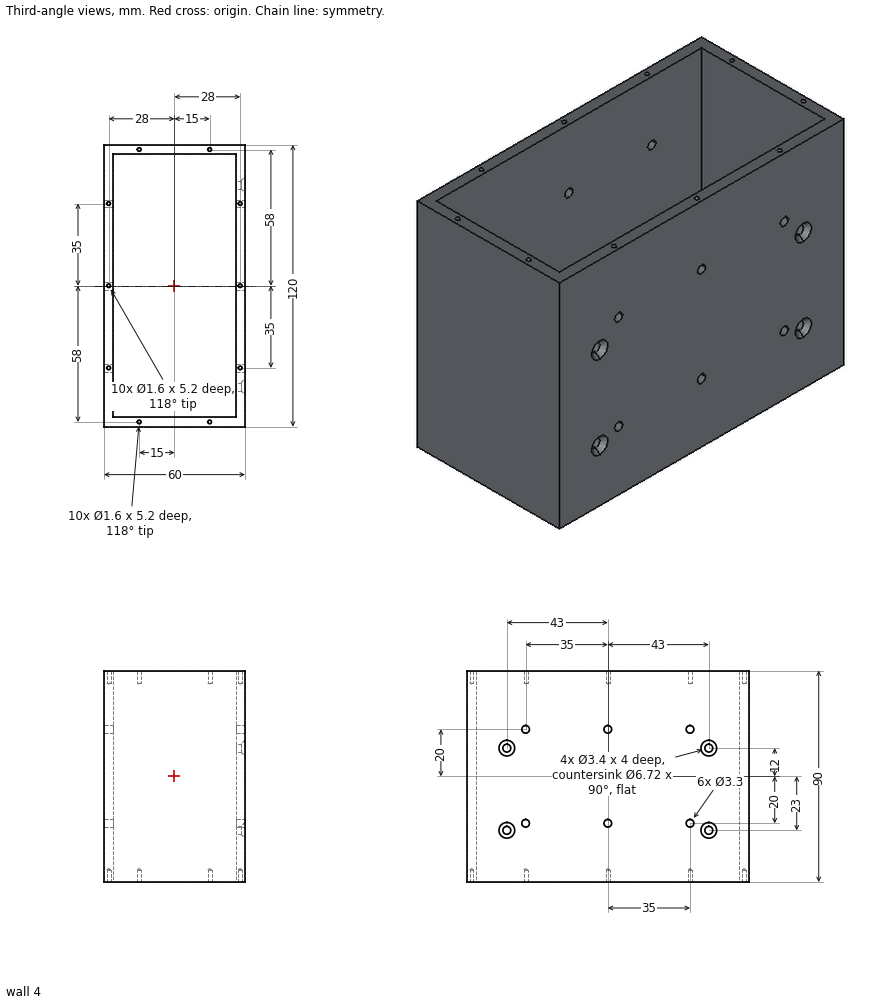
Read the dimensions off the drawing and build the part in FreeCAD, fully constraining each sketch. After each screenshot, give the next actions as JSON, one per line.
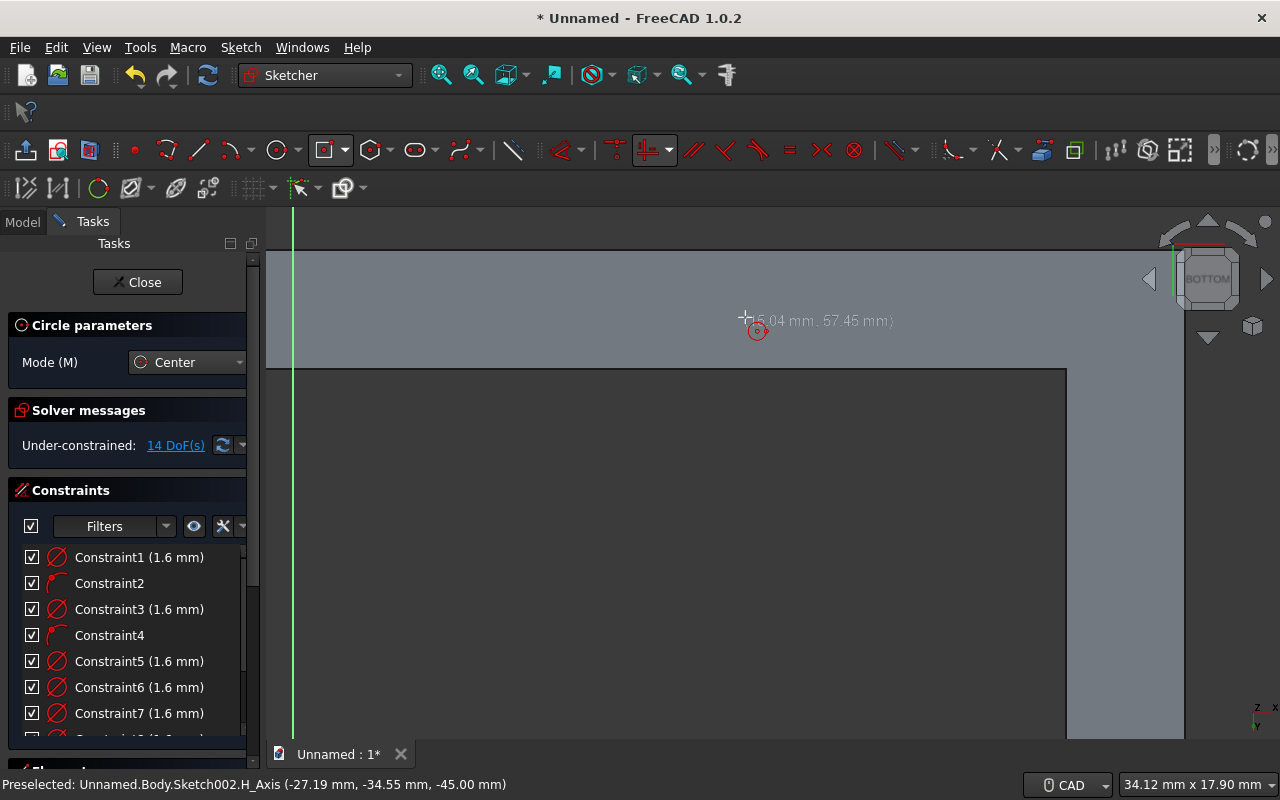
{"action": "scroll", "coordinate": [746, 317], "scroll_direction": "down", "scroll_amount": 12}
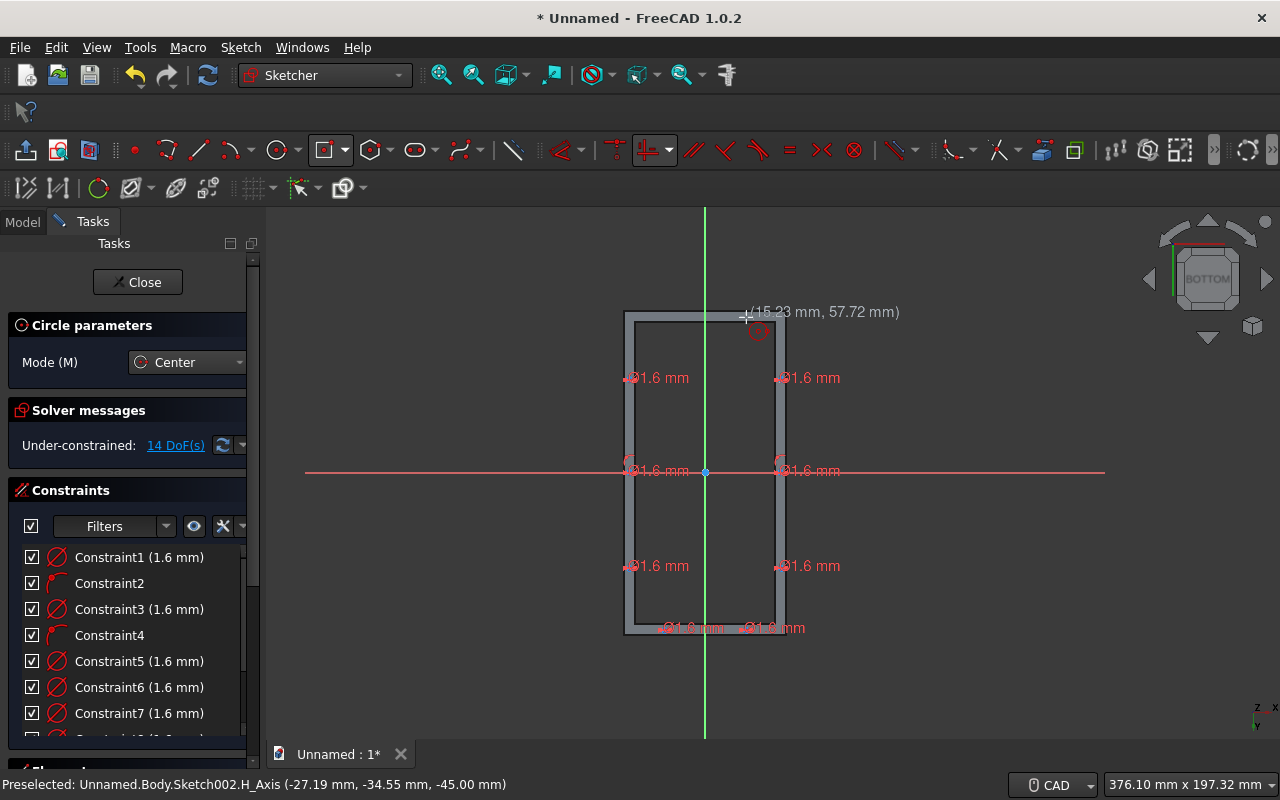
{"action": "left_click", "coordinate": [746, 317]}
{"action": "mouse_move", "coordinate": [747, 315]}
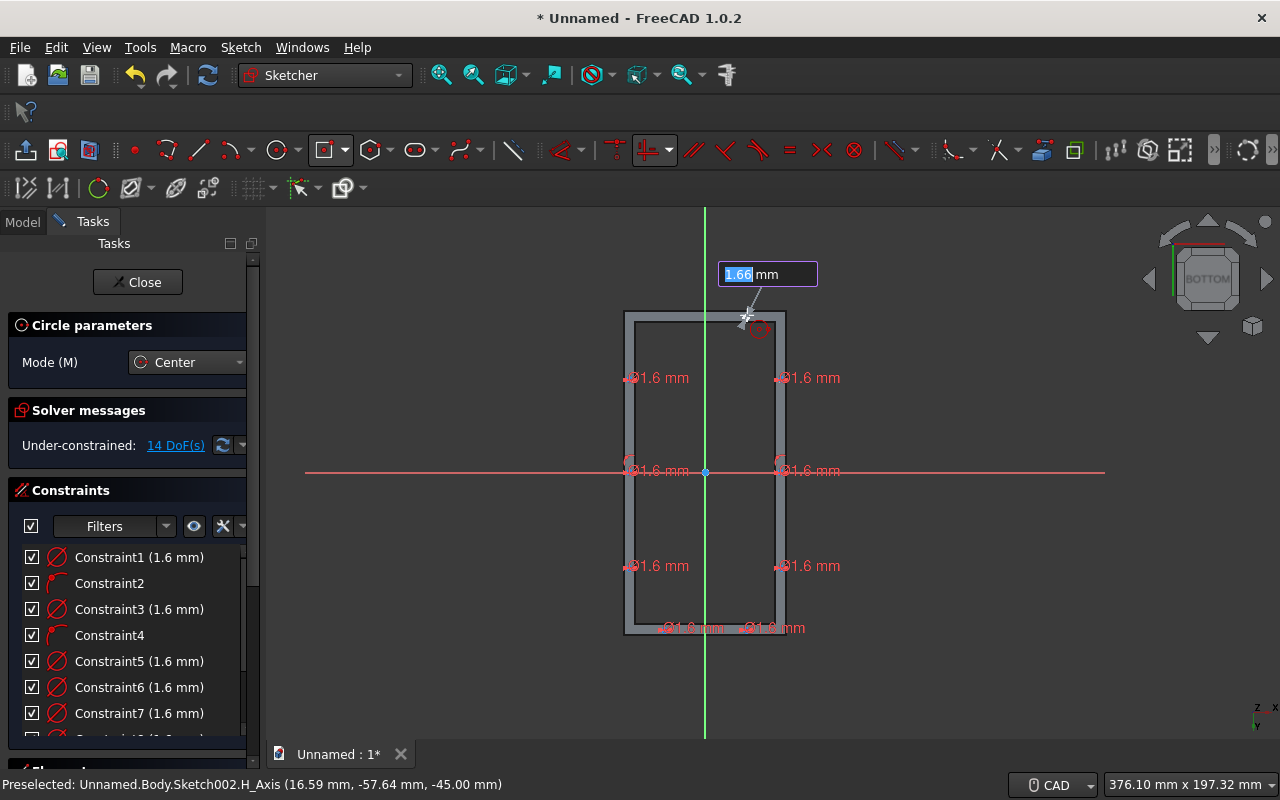
{"action": "type", "text": "1.6"}
{"action": "key", "text": "Return"}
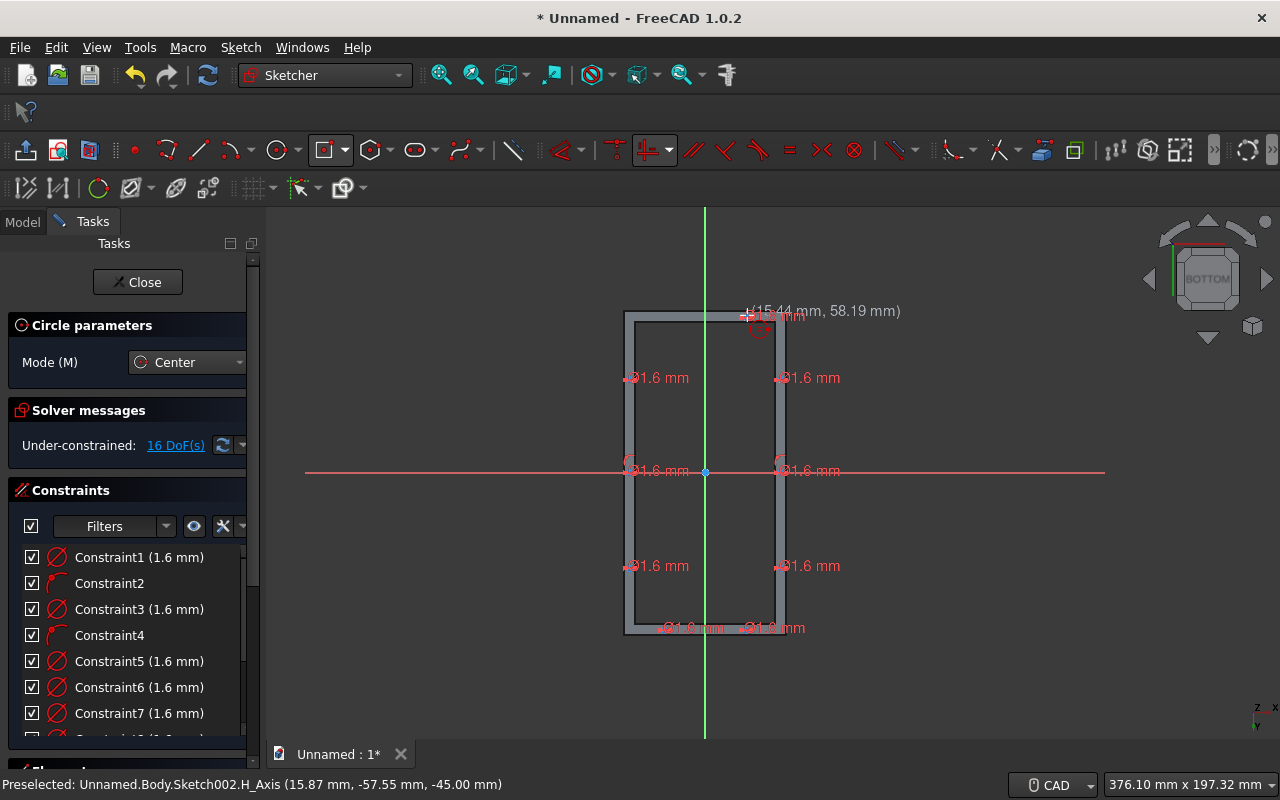
{"action": "scroll", "coordinate": [665, 317], "scroll_direction": "up", "scroll_amount": 12}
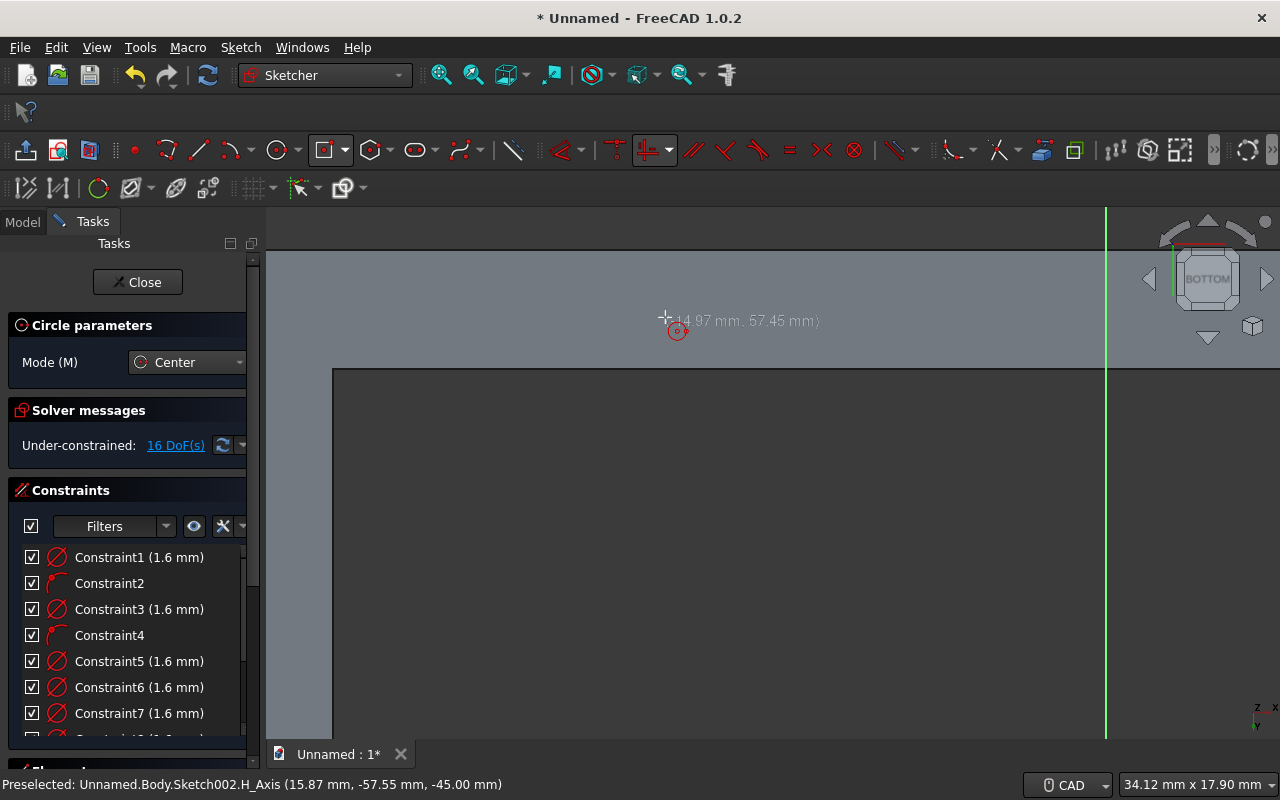
{"action": "scroll", "coordinate": [664, 317], "scroll_direction": "down", "scroll_amount": 12}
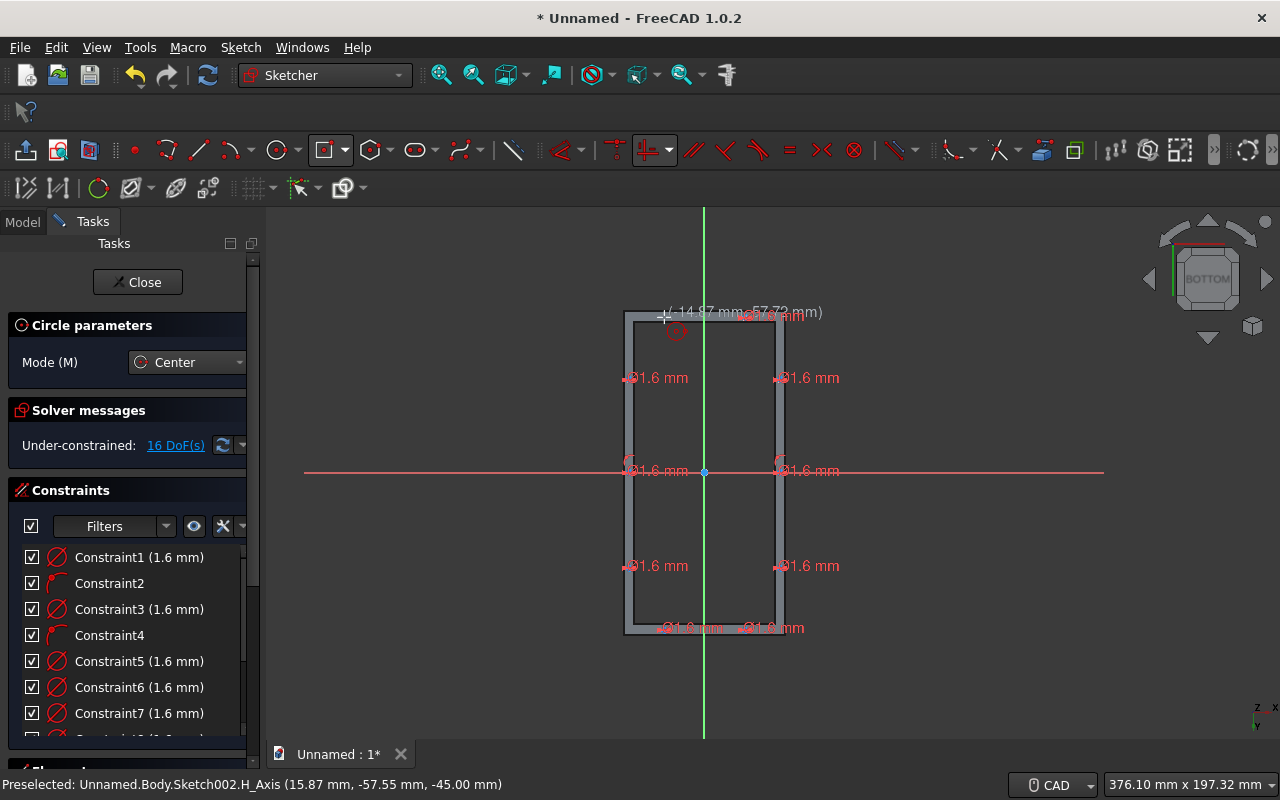
{"action": "left_click", "coordinate": [664, 317]}
{"action": "mouse_move", "coordinate": [666, 315]}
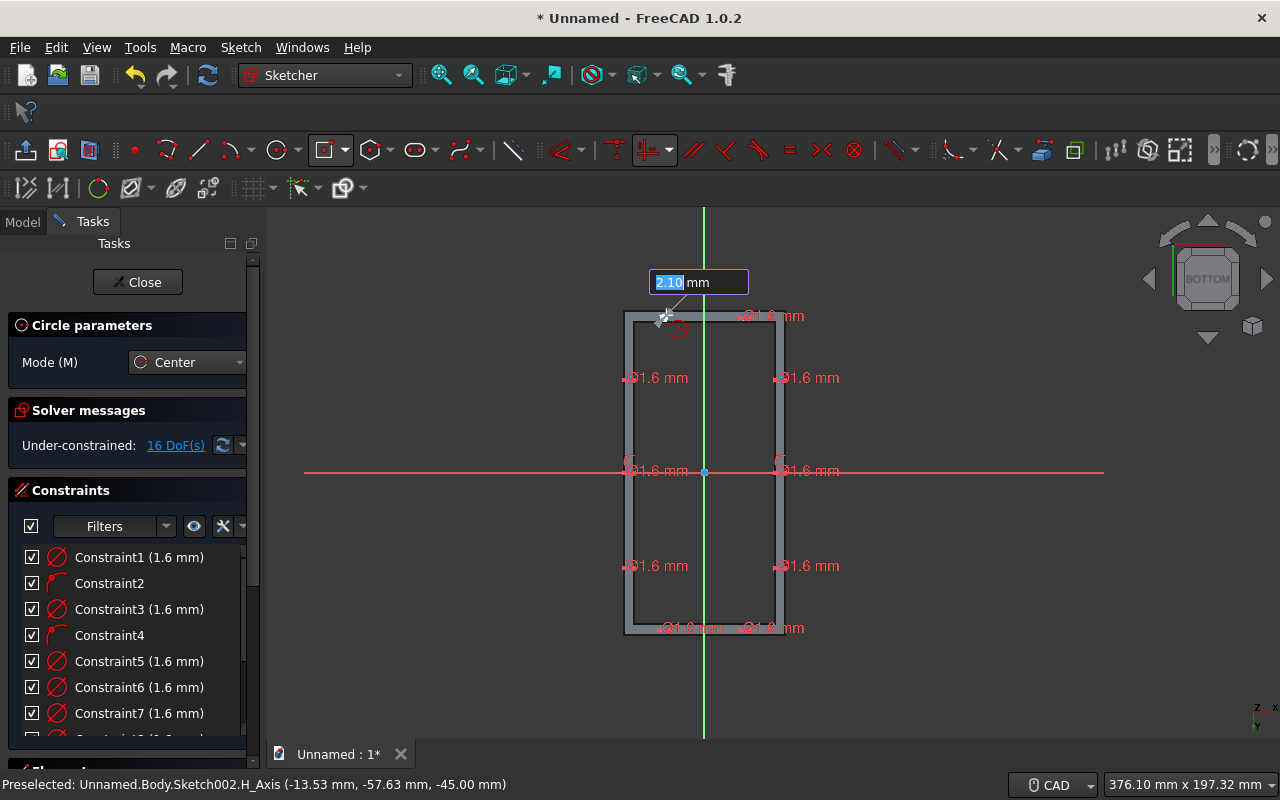
{"action": "type", "text": "1.6"}
{"action": "key", "text": "Return"}
{"action": "key", "text": "Escape"}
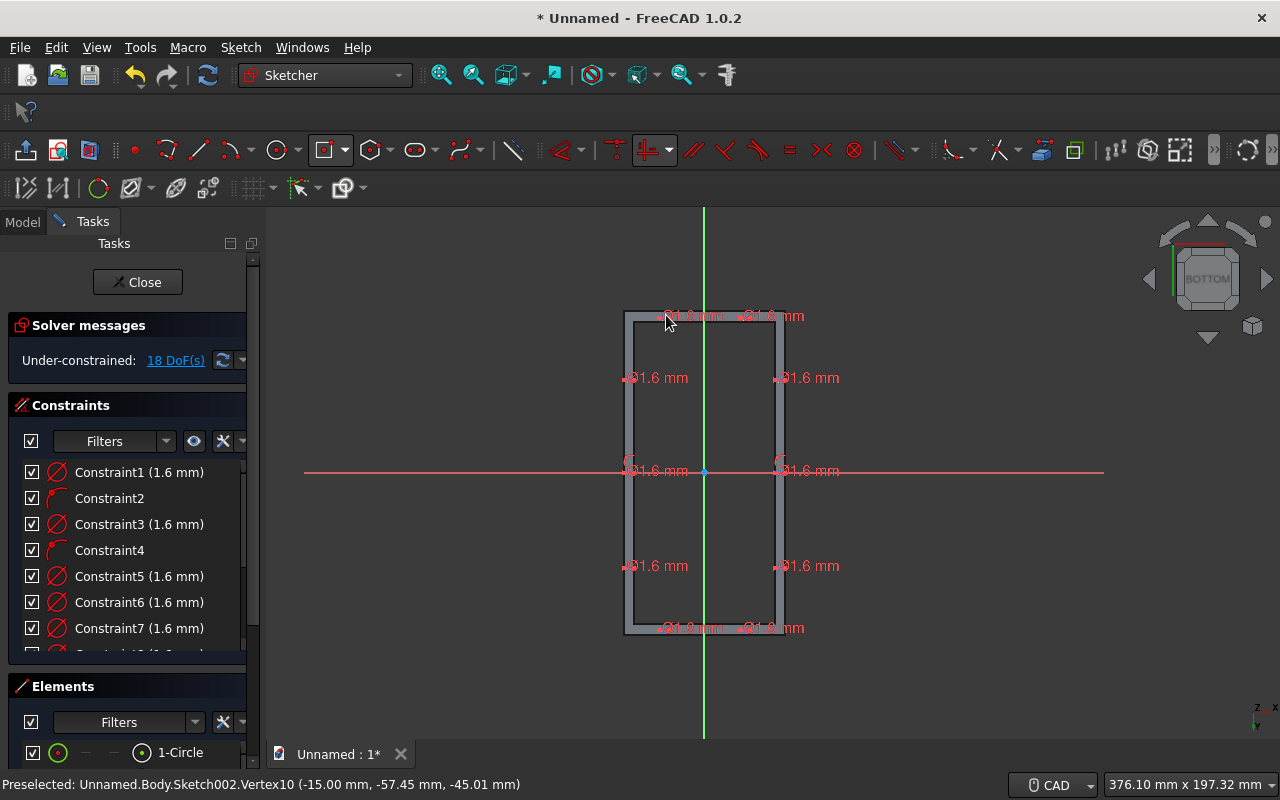
{"action": "left_click", "coordinate": [745, 630]}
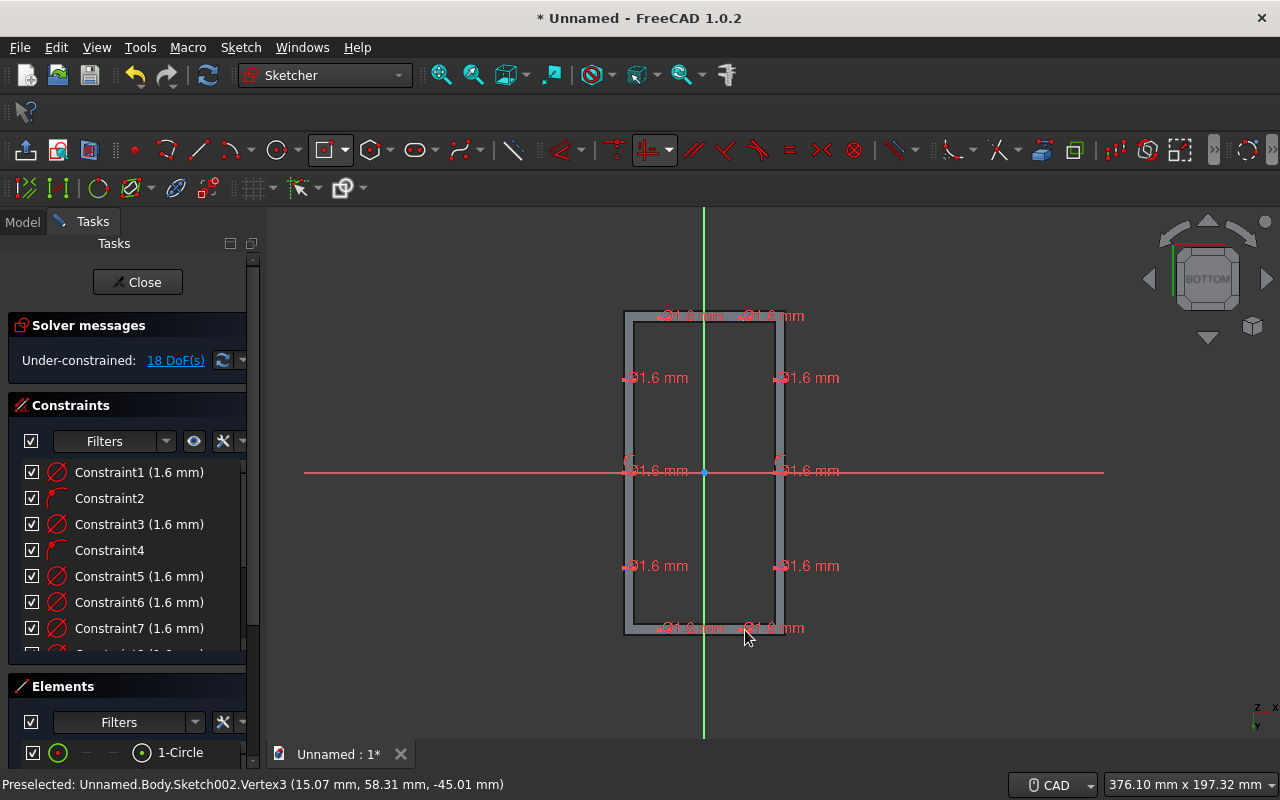
{"action": "left_click", "coordinate": [664, 630]}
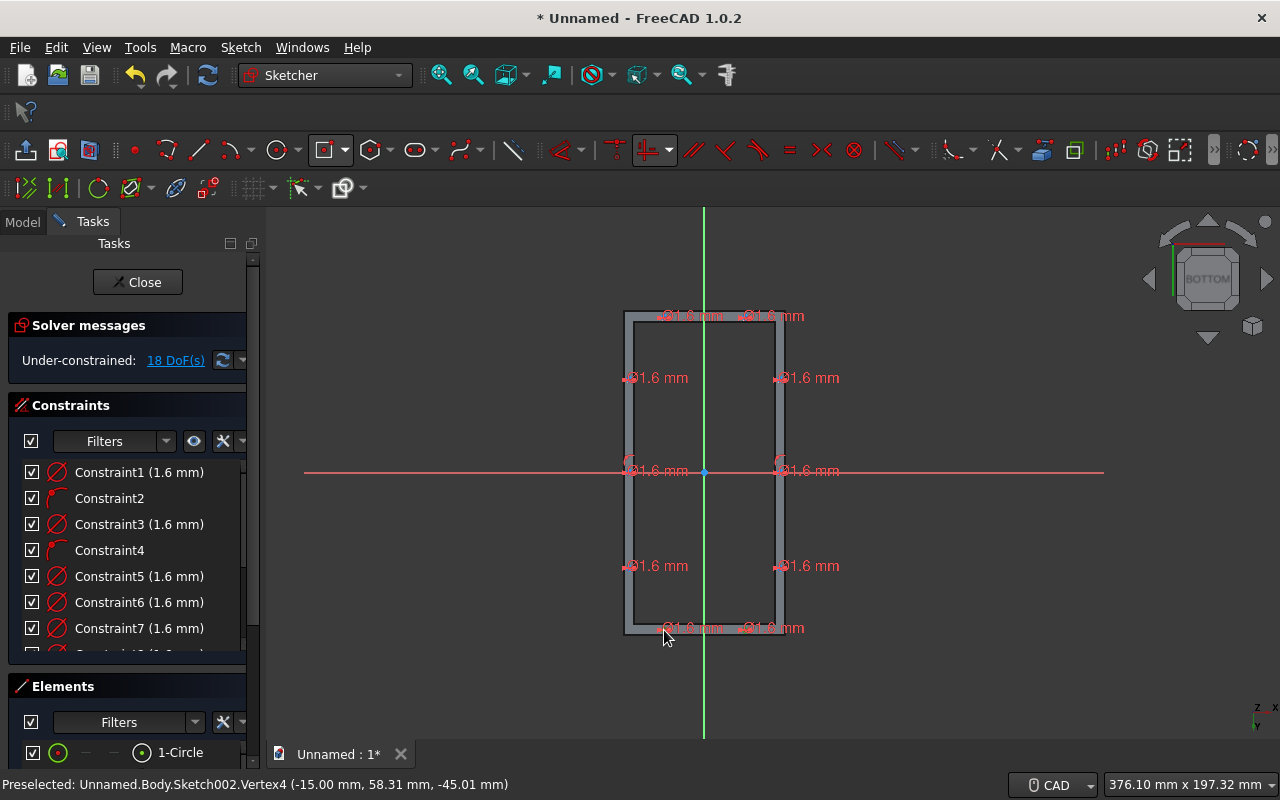
{"action": "left_click", "coordinate": [672, 150]}